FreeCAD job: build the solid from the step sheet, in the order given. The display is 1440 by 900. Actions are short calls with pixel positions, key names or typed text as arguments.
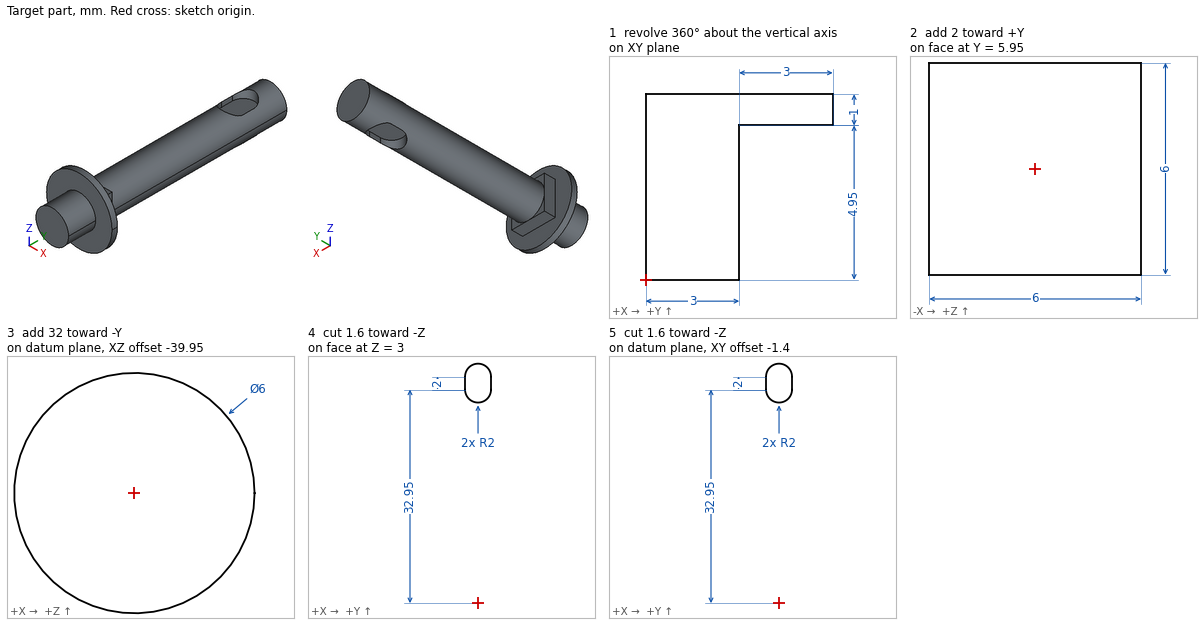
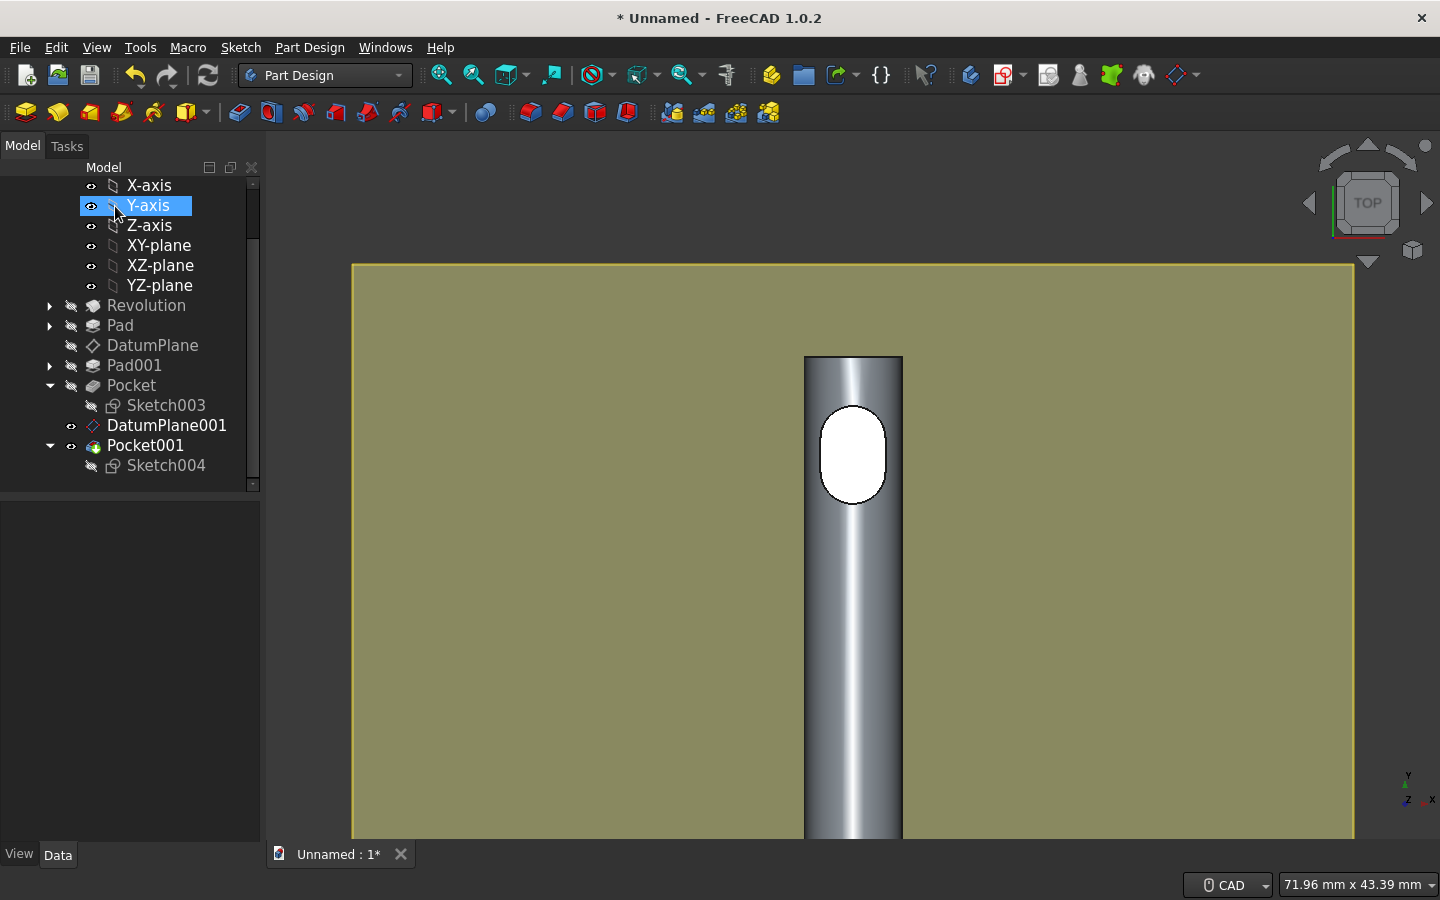
click(116, 426)
key(space)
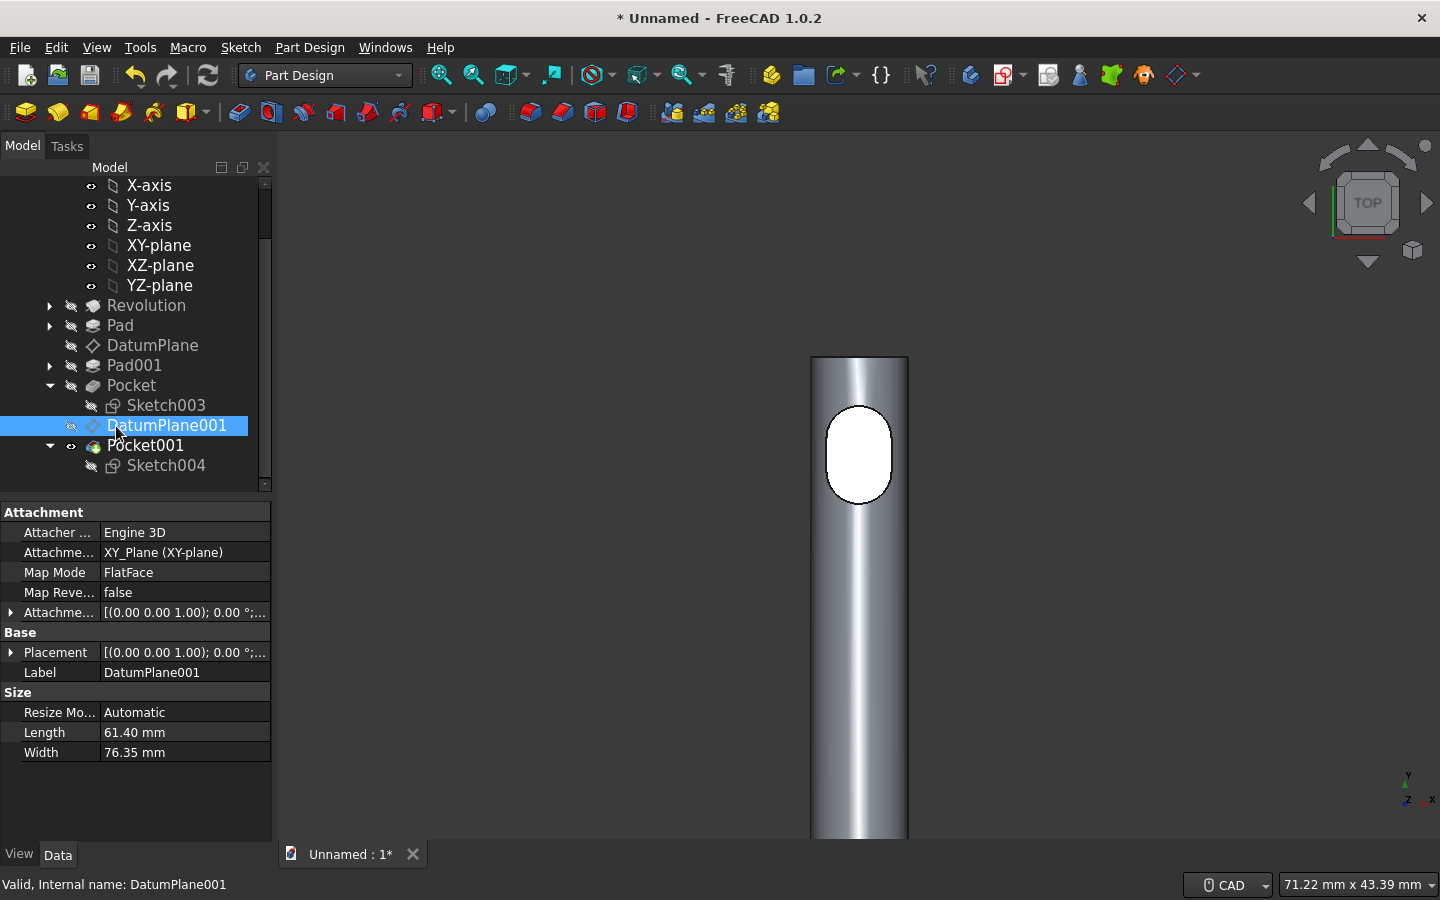
key(0)